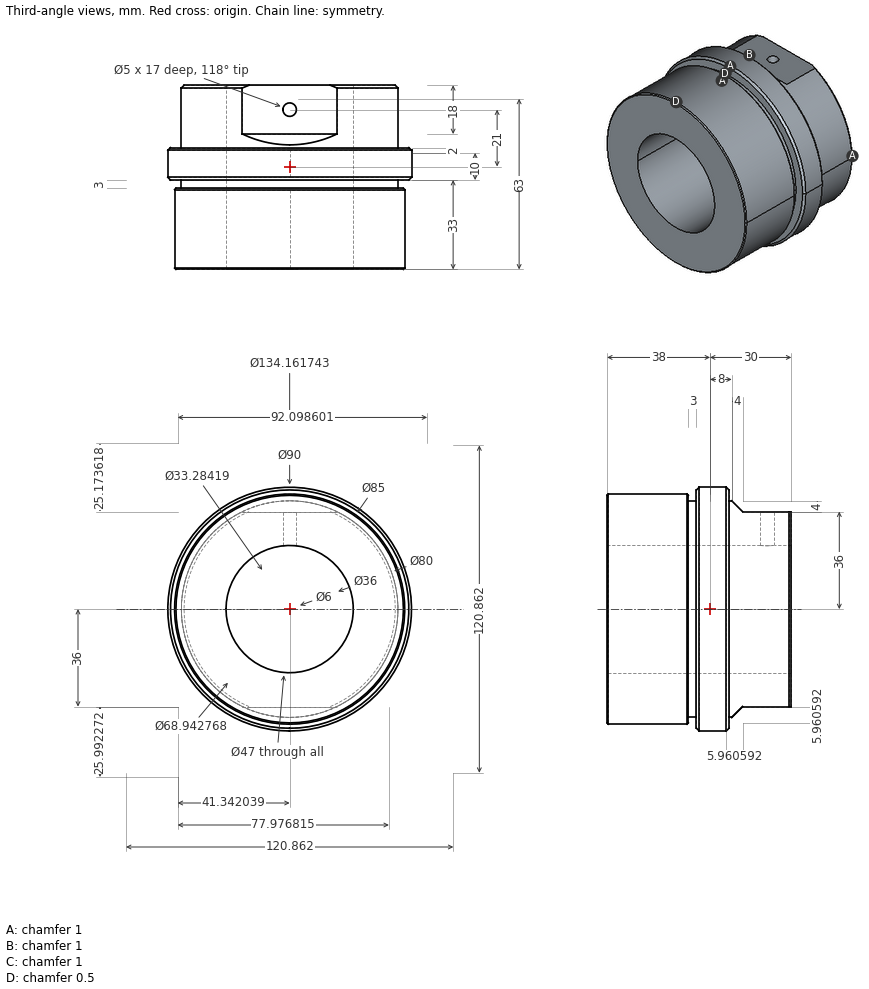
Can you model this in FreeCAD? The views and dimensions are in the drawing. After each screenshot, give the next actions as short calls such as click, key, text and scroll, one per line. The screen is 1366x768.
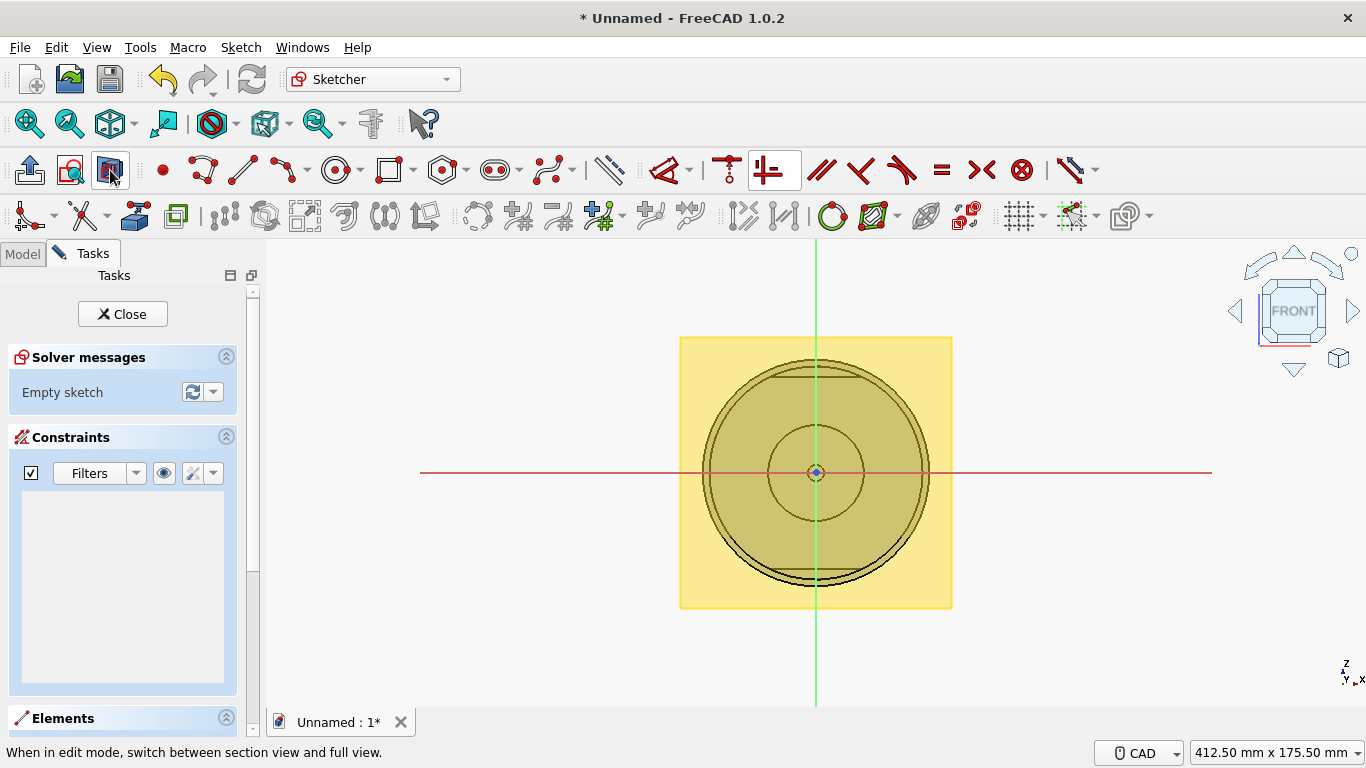
click(336, 170)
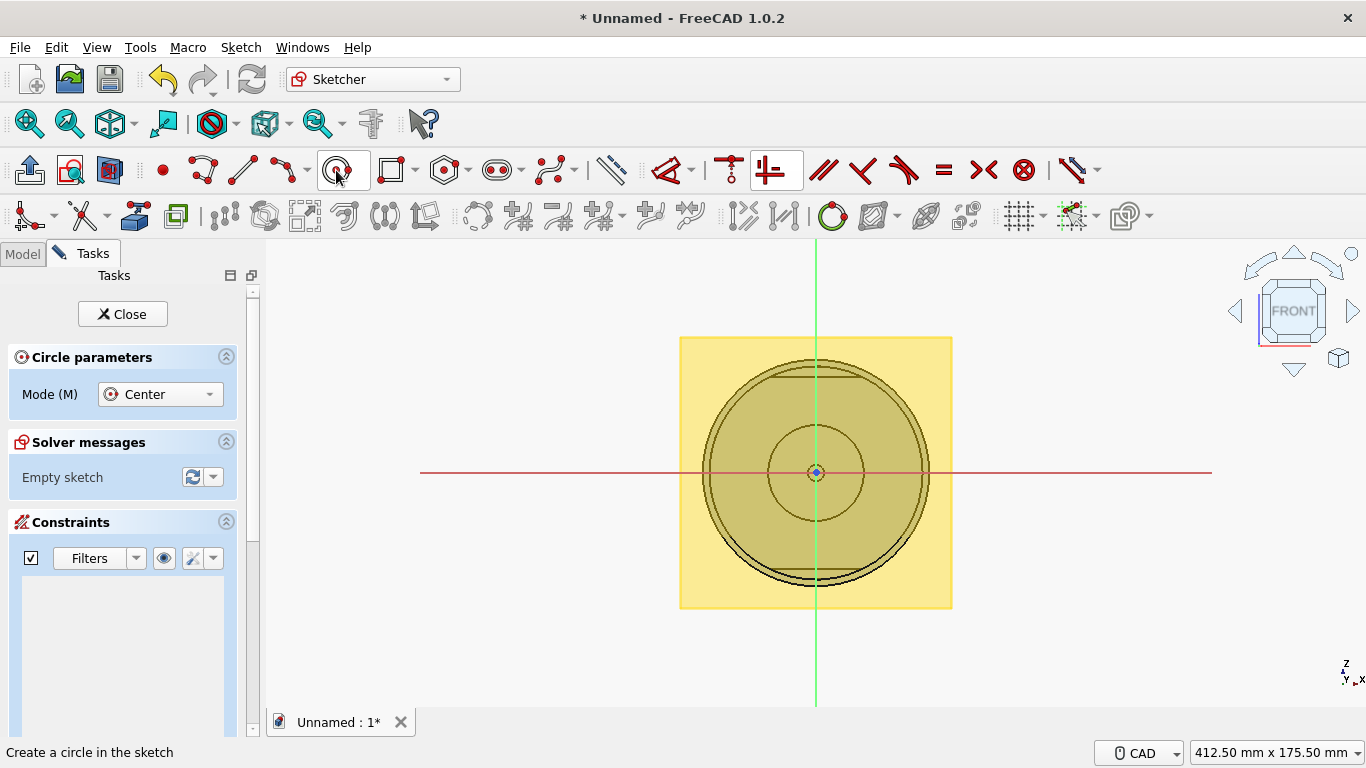
click(816, 473)
click(901, 388)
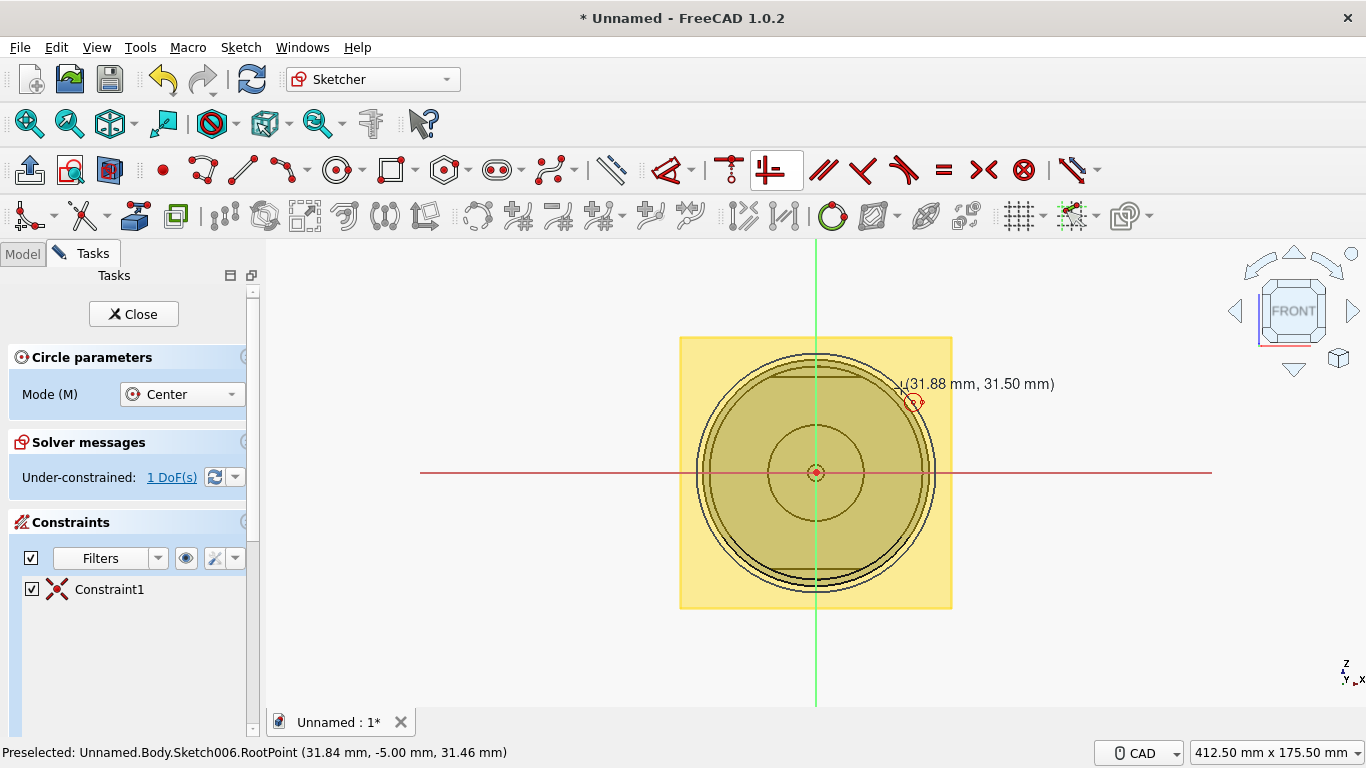
click(816, 473)
click(847, 442)
key(Escape)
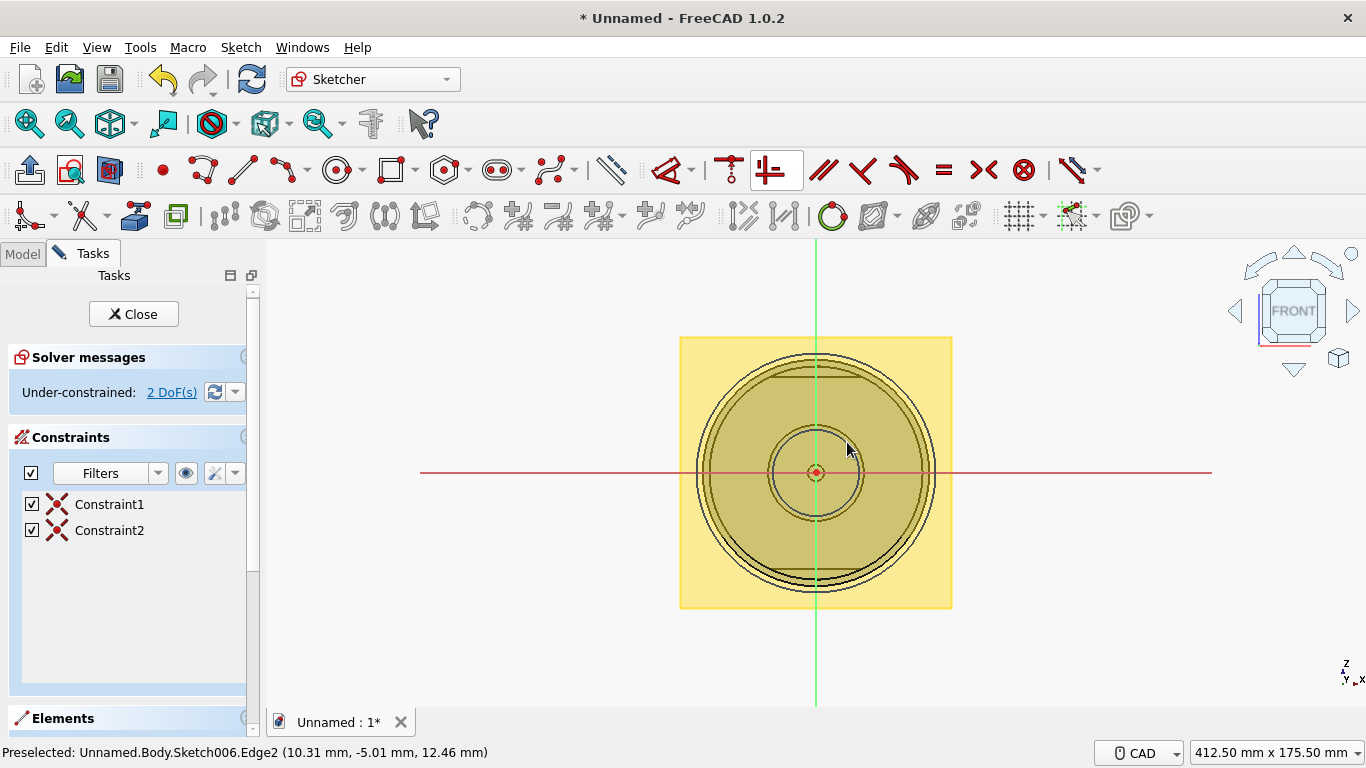
click(666, 170)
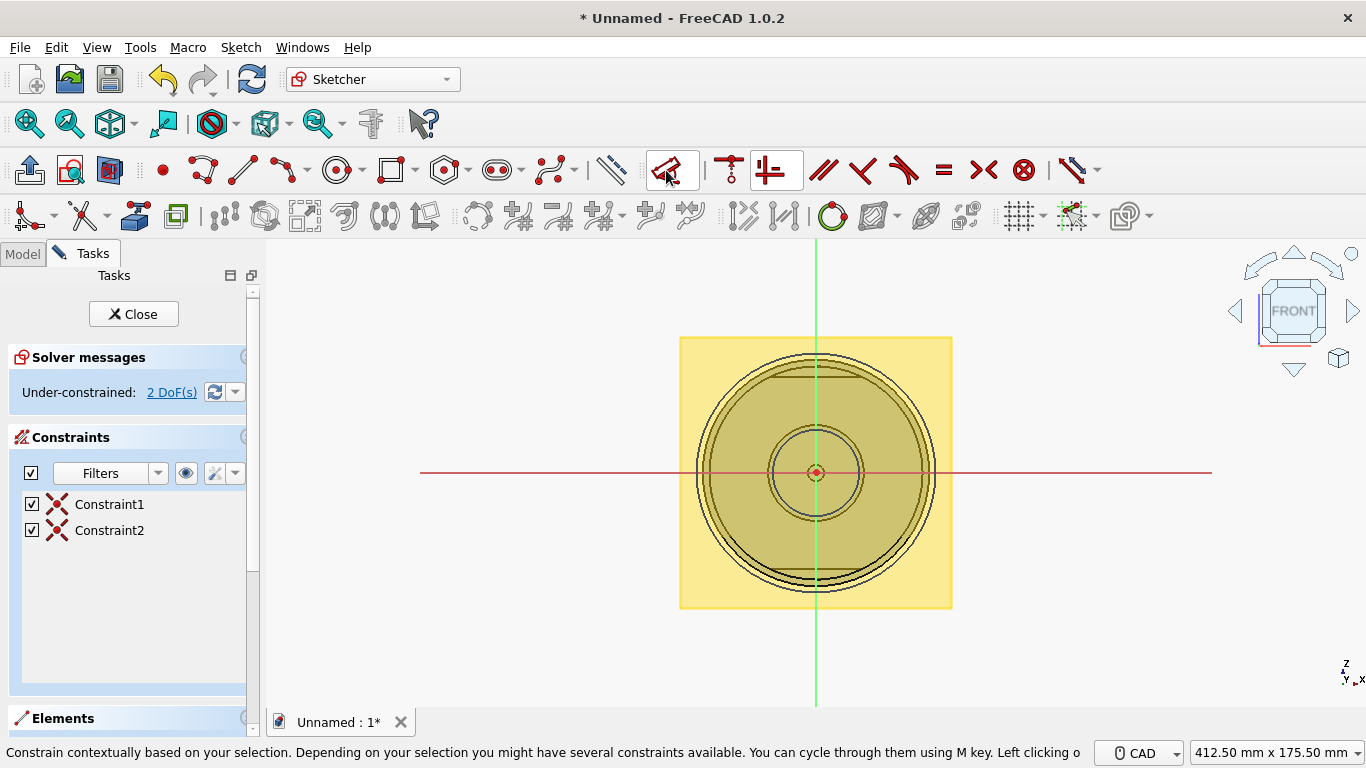
click(900, 388)
click(922, 365)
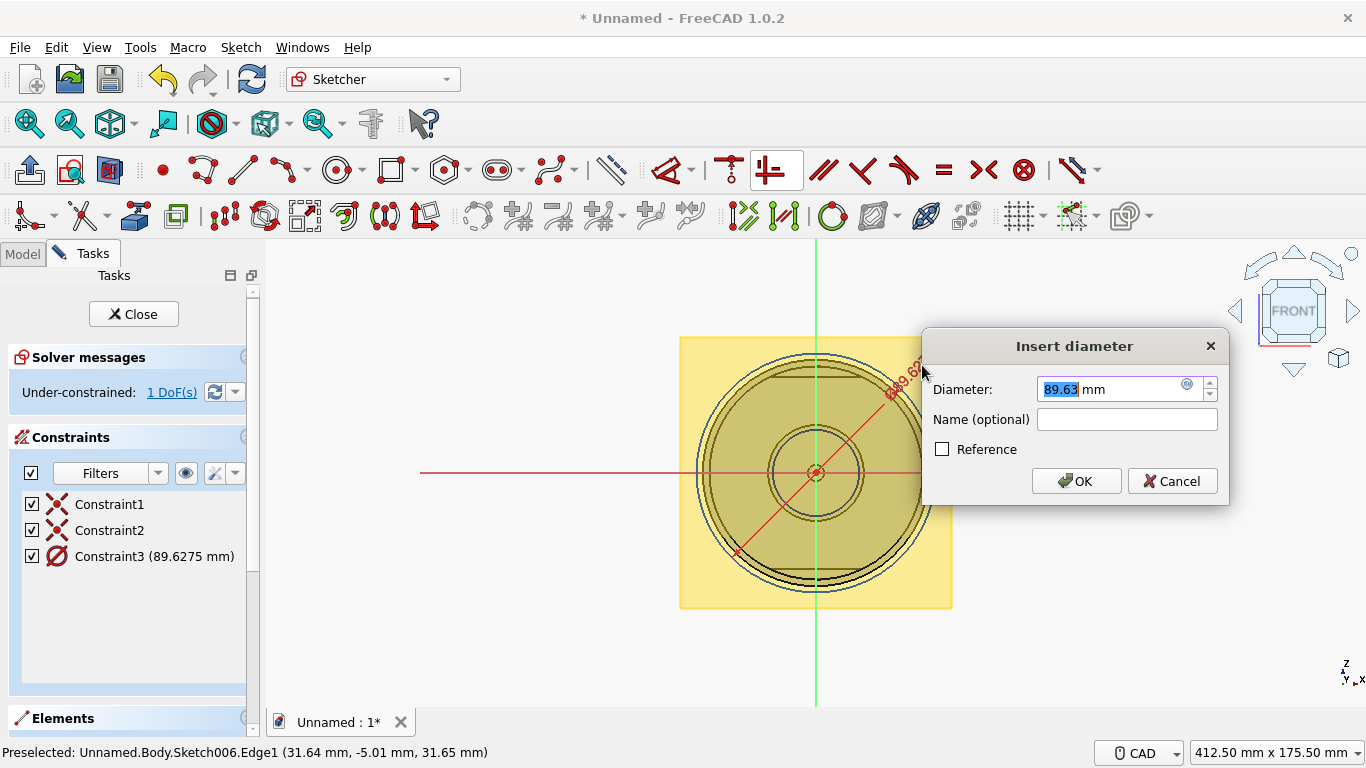
text(90)
key(Return)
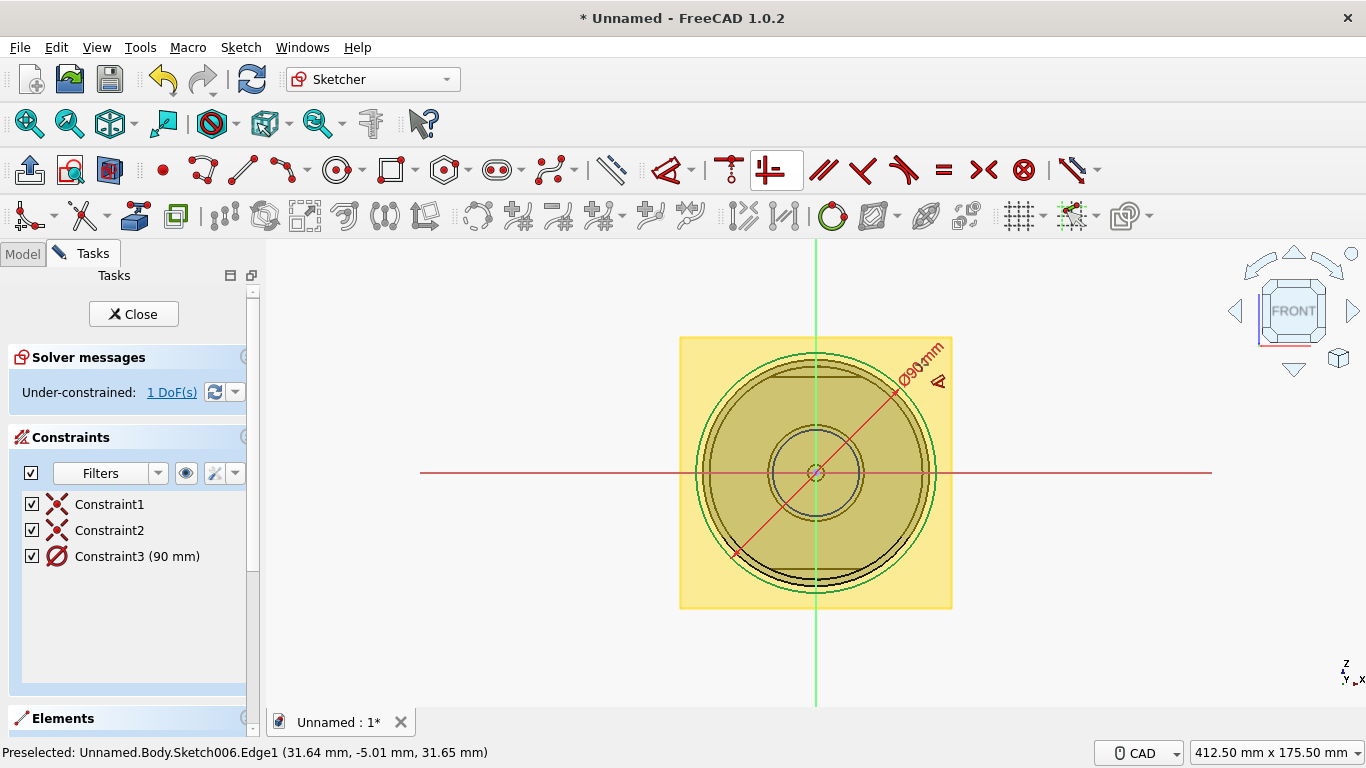
click(846, 442)
click(868, 419)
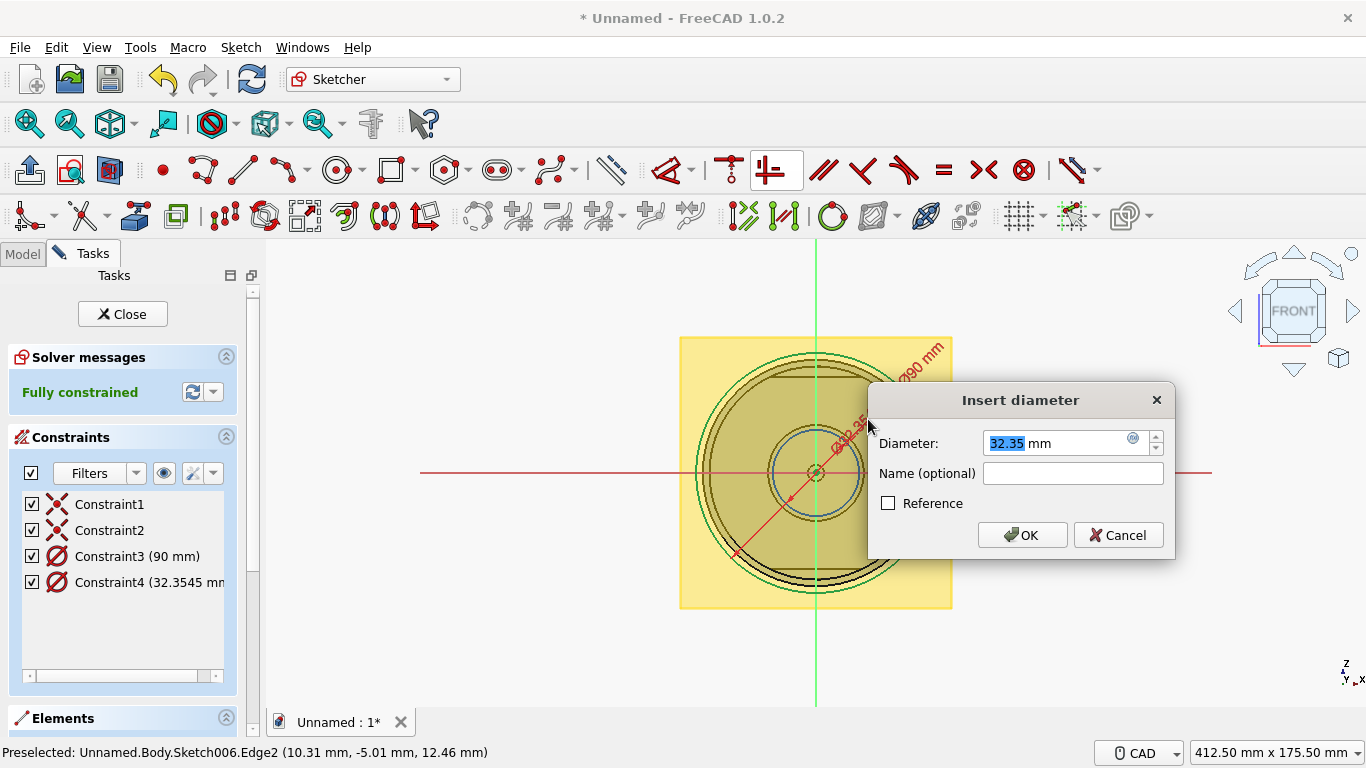
text(33.28419)
key(Return)
key(Escape)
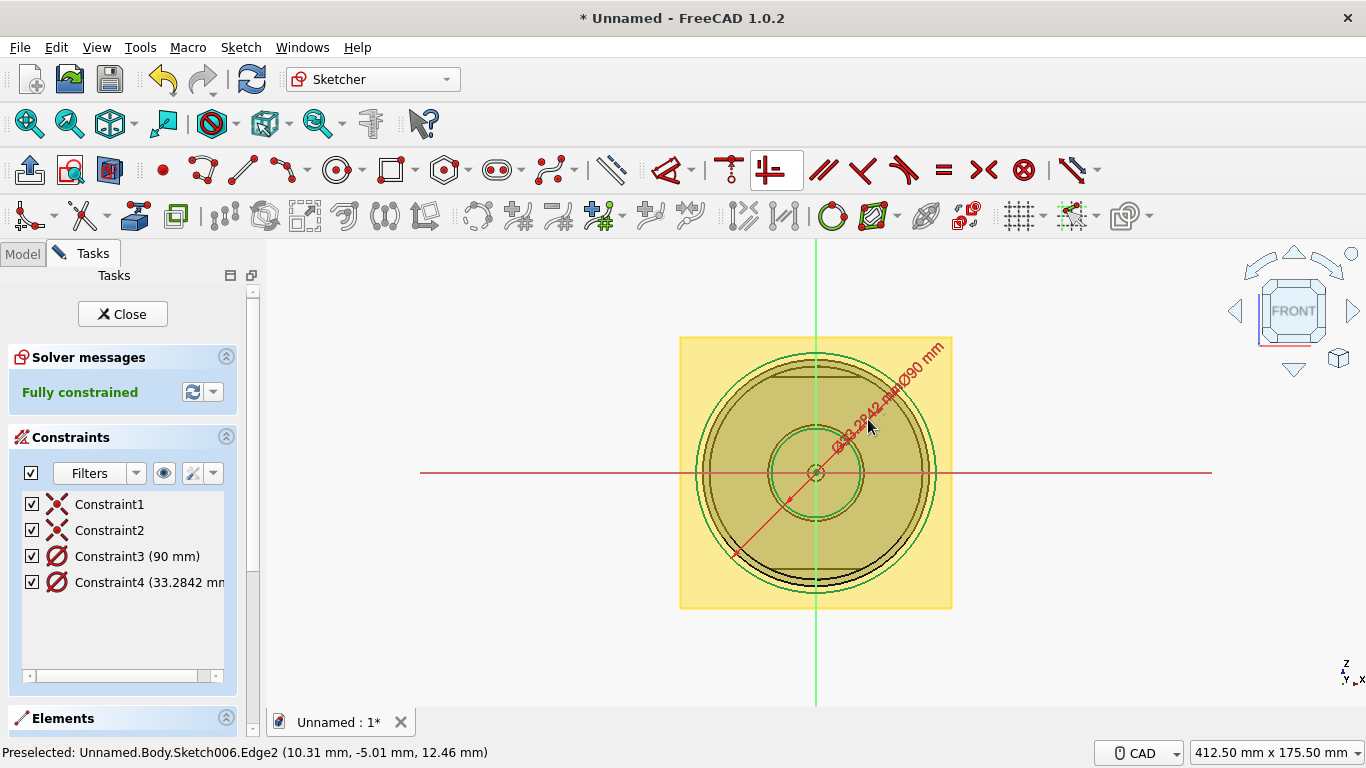
click(123, 314)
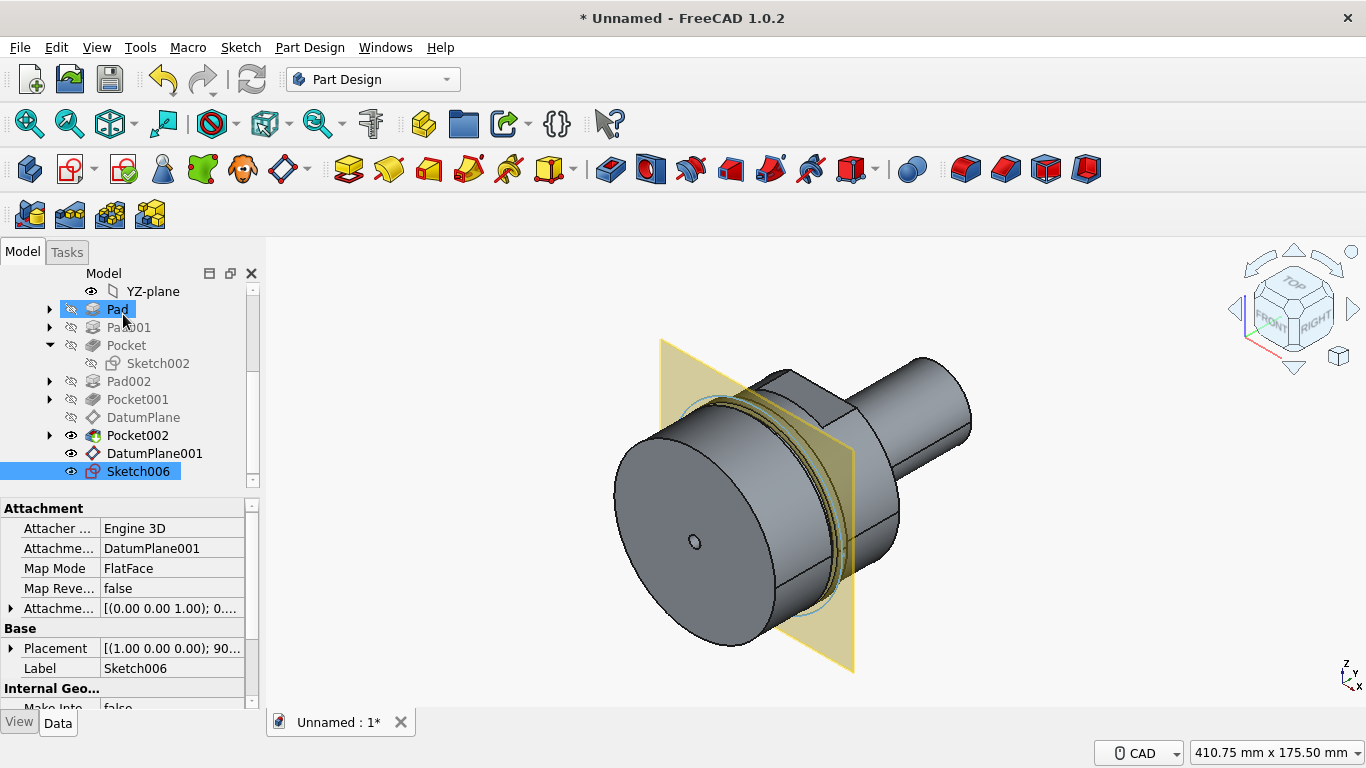
click(350, 170)